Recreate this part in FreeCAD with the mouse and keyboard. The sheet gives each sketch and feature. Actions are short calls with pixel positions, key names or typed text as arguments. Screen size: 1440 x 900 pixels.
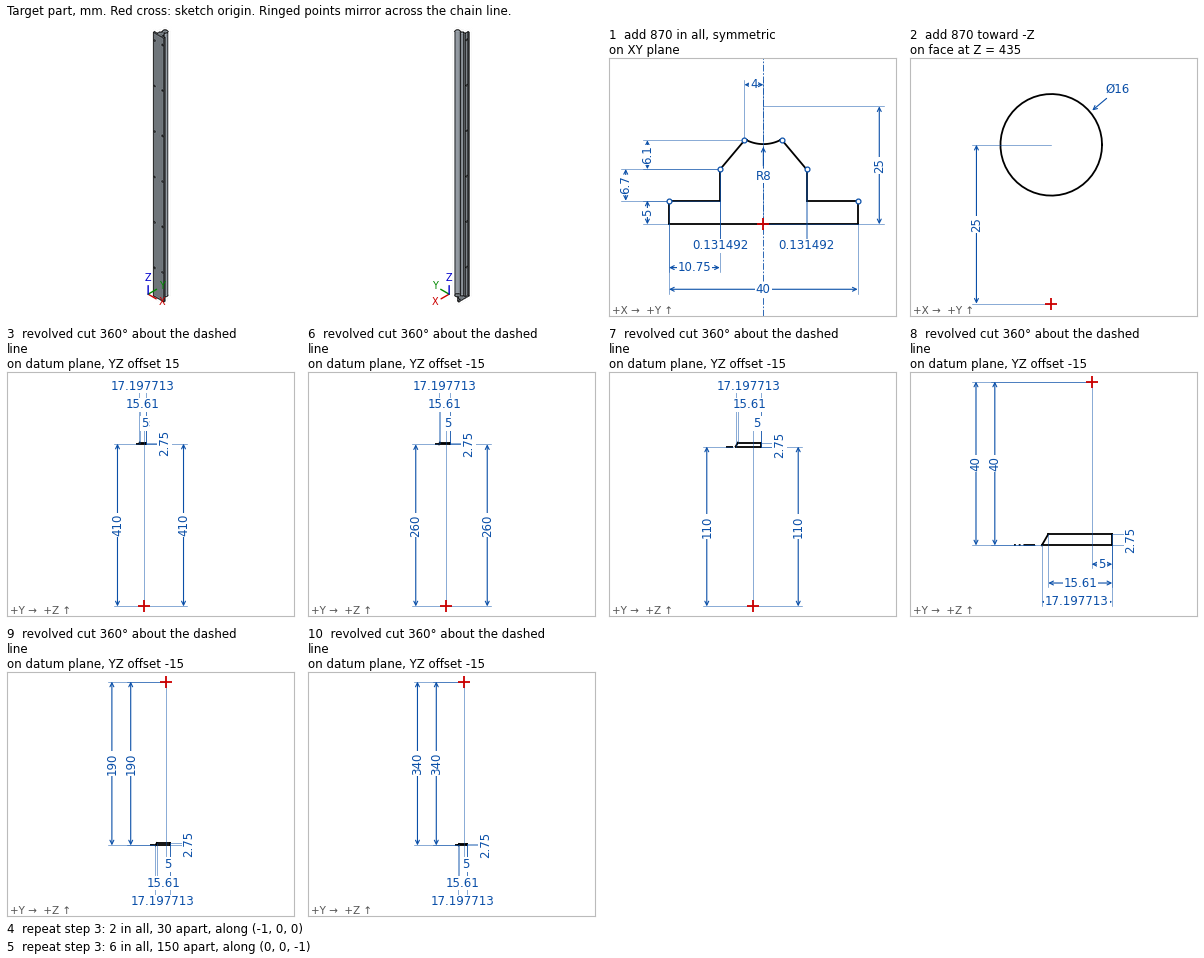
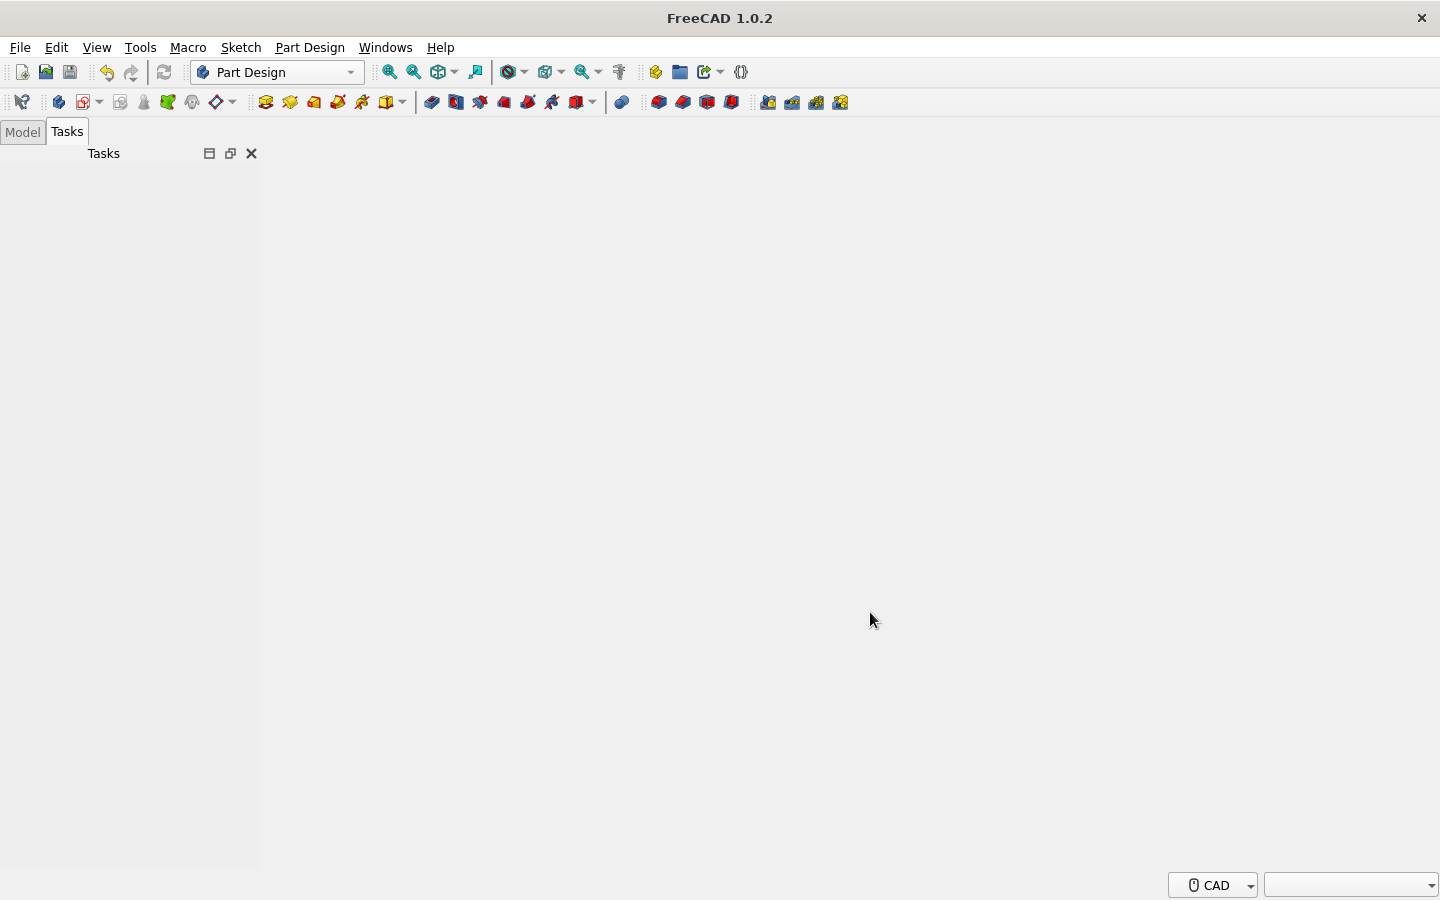
click(22, 72)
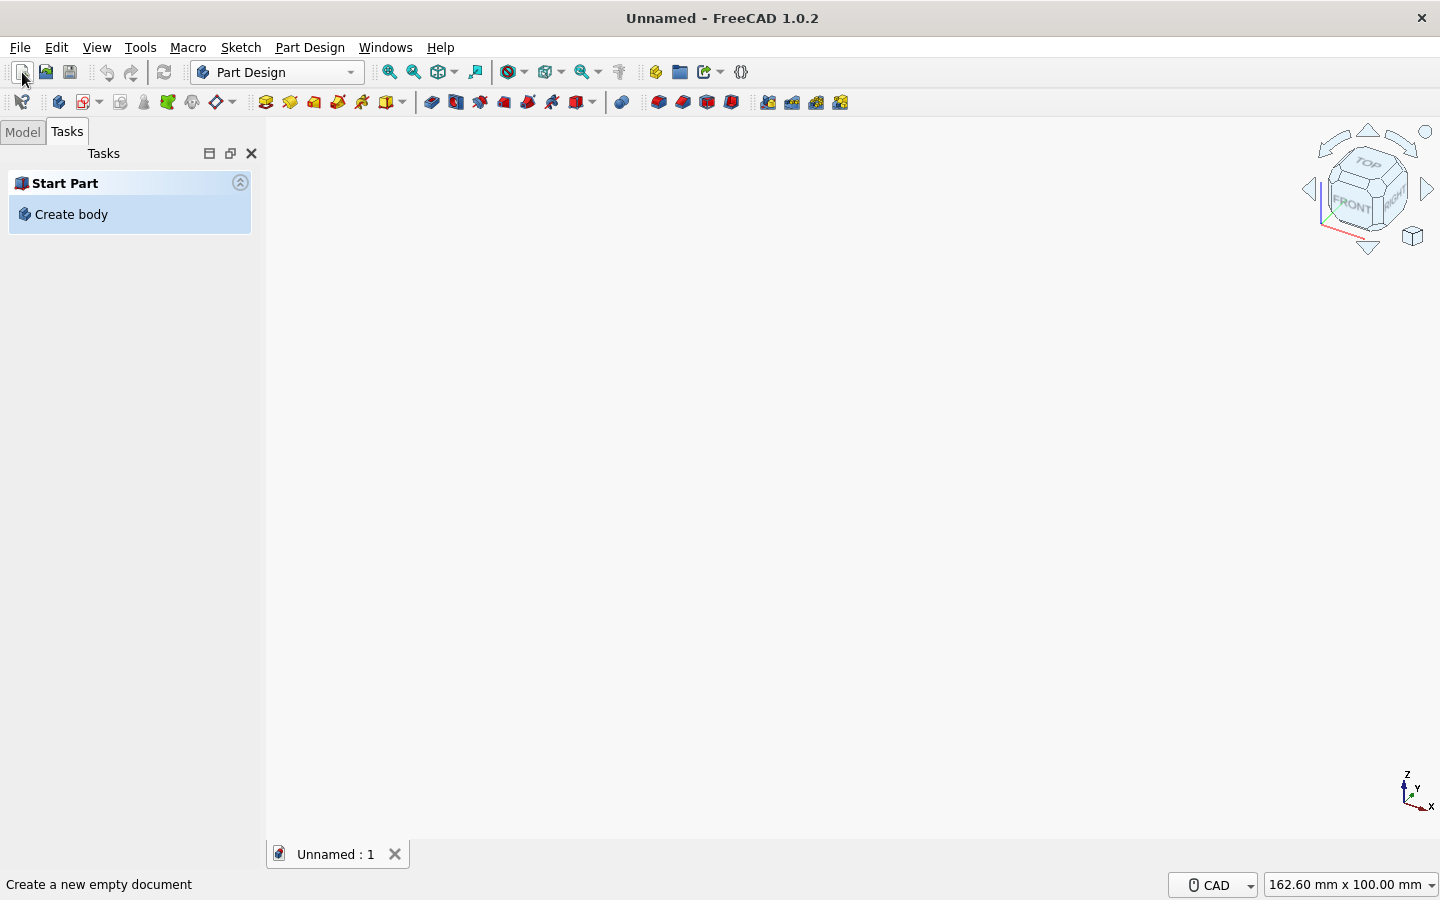
click(84, 102)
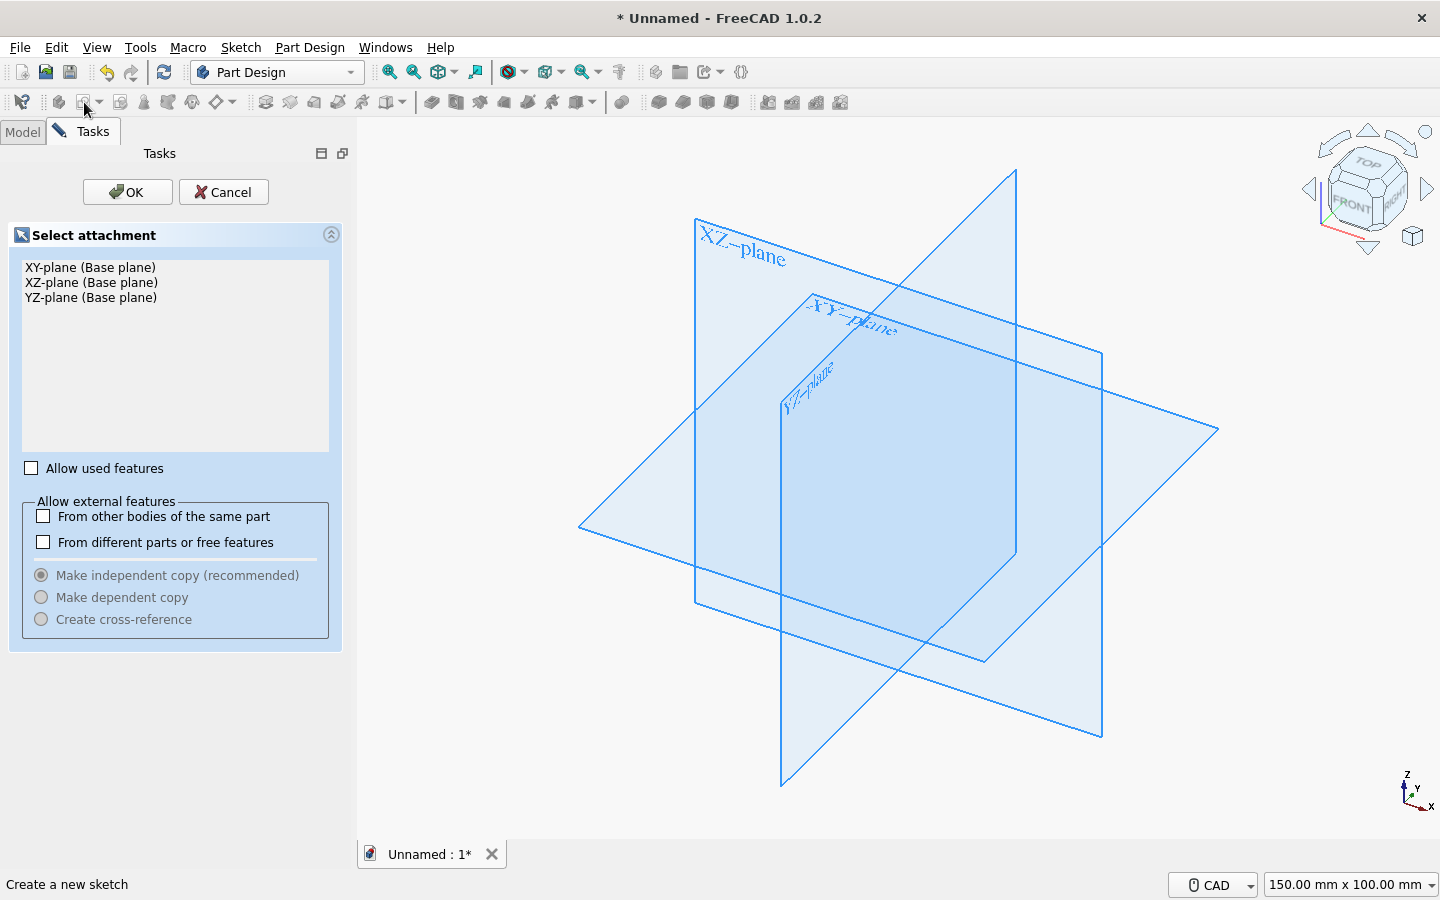
click(82, 268)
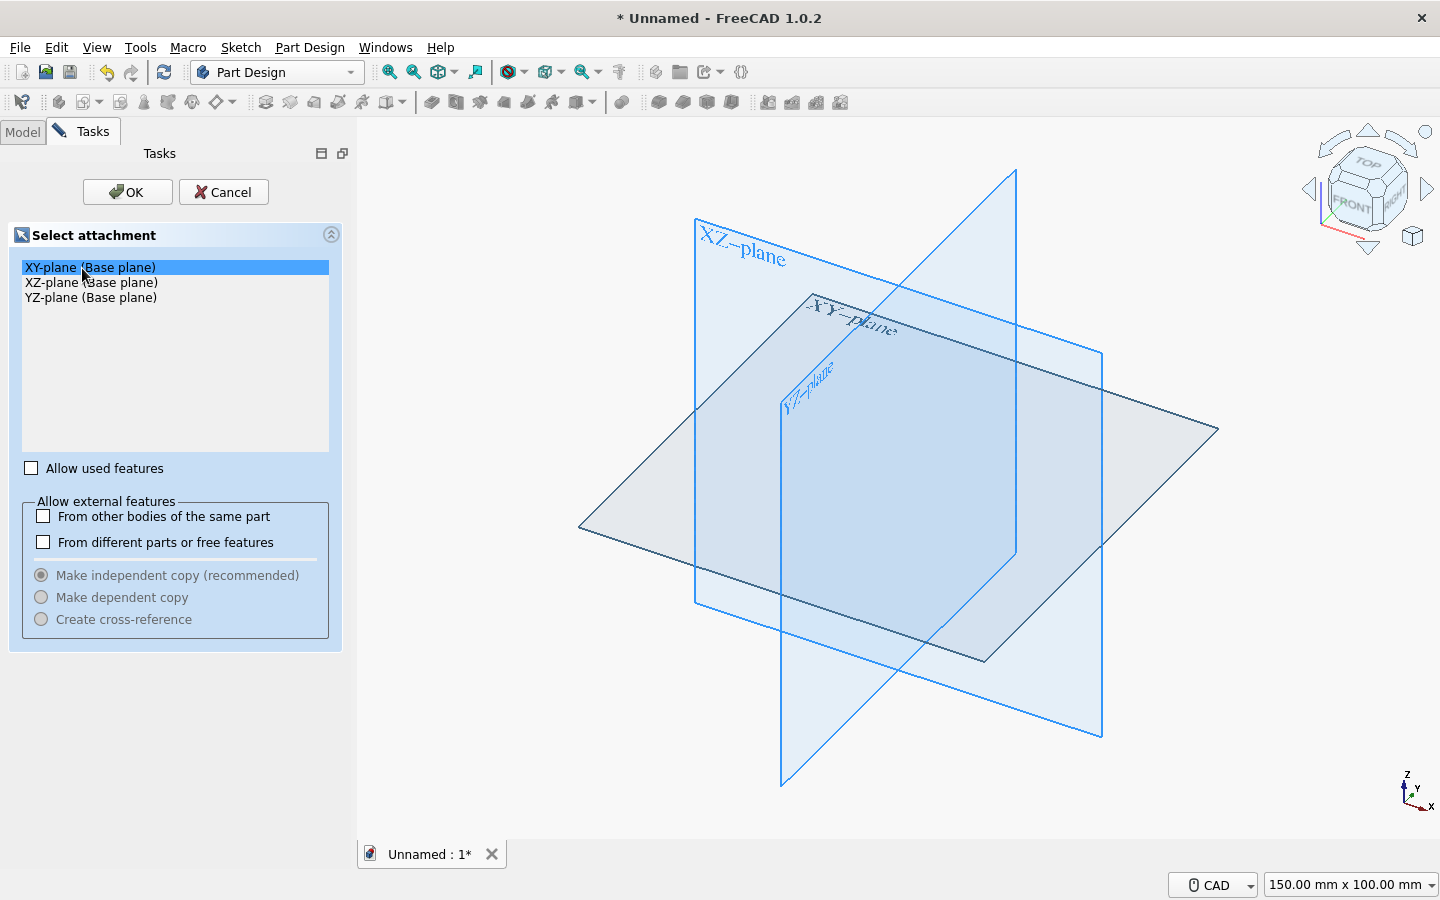
click(128, 192)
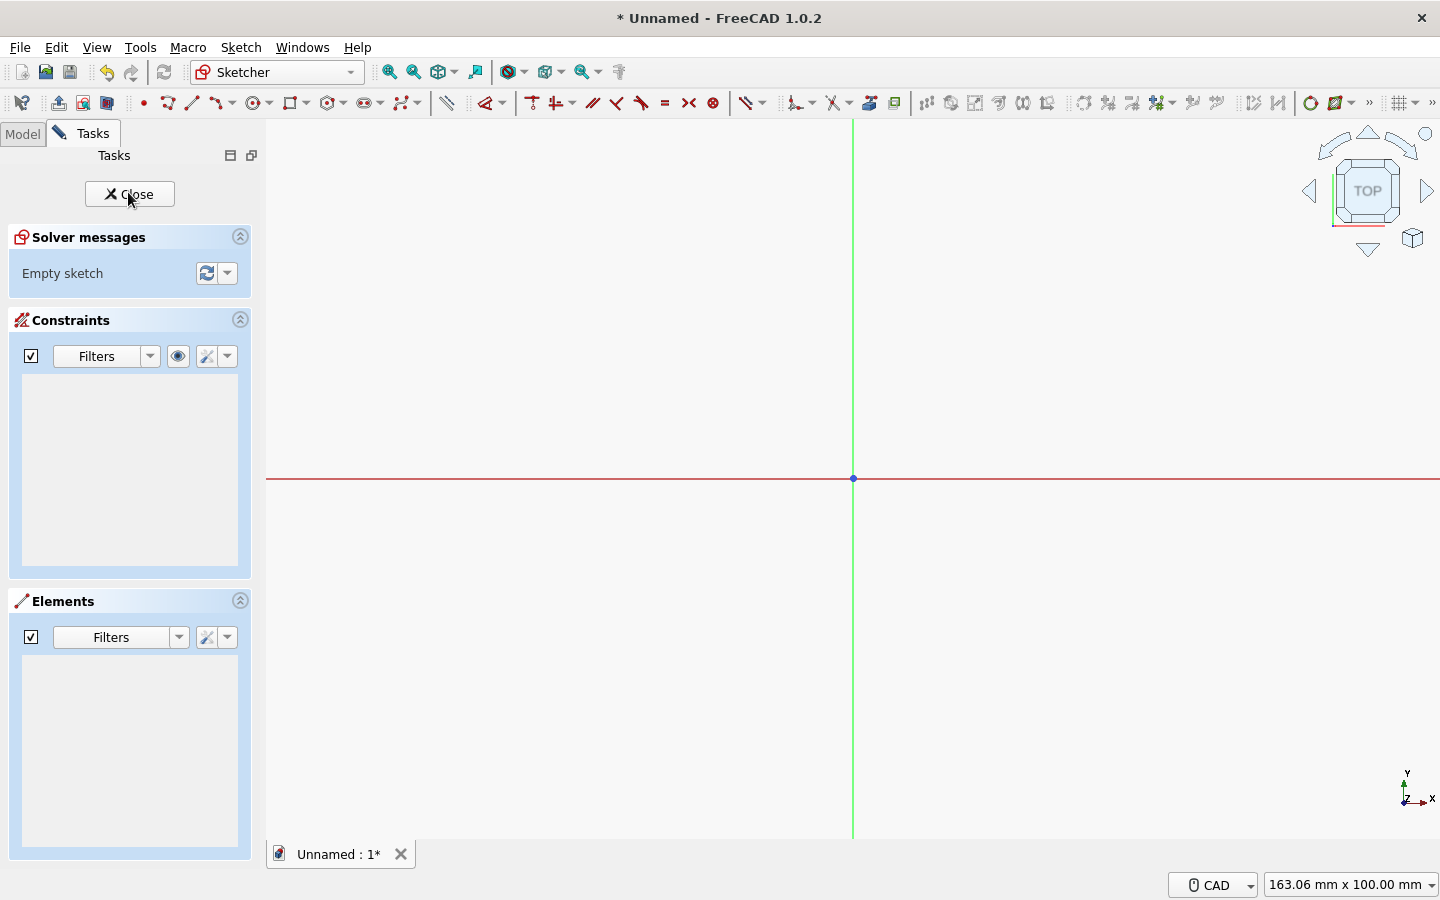
scroll(909, 363, up, 4)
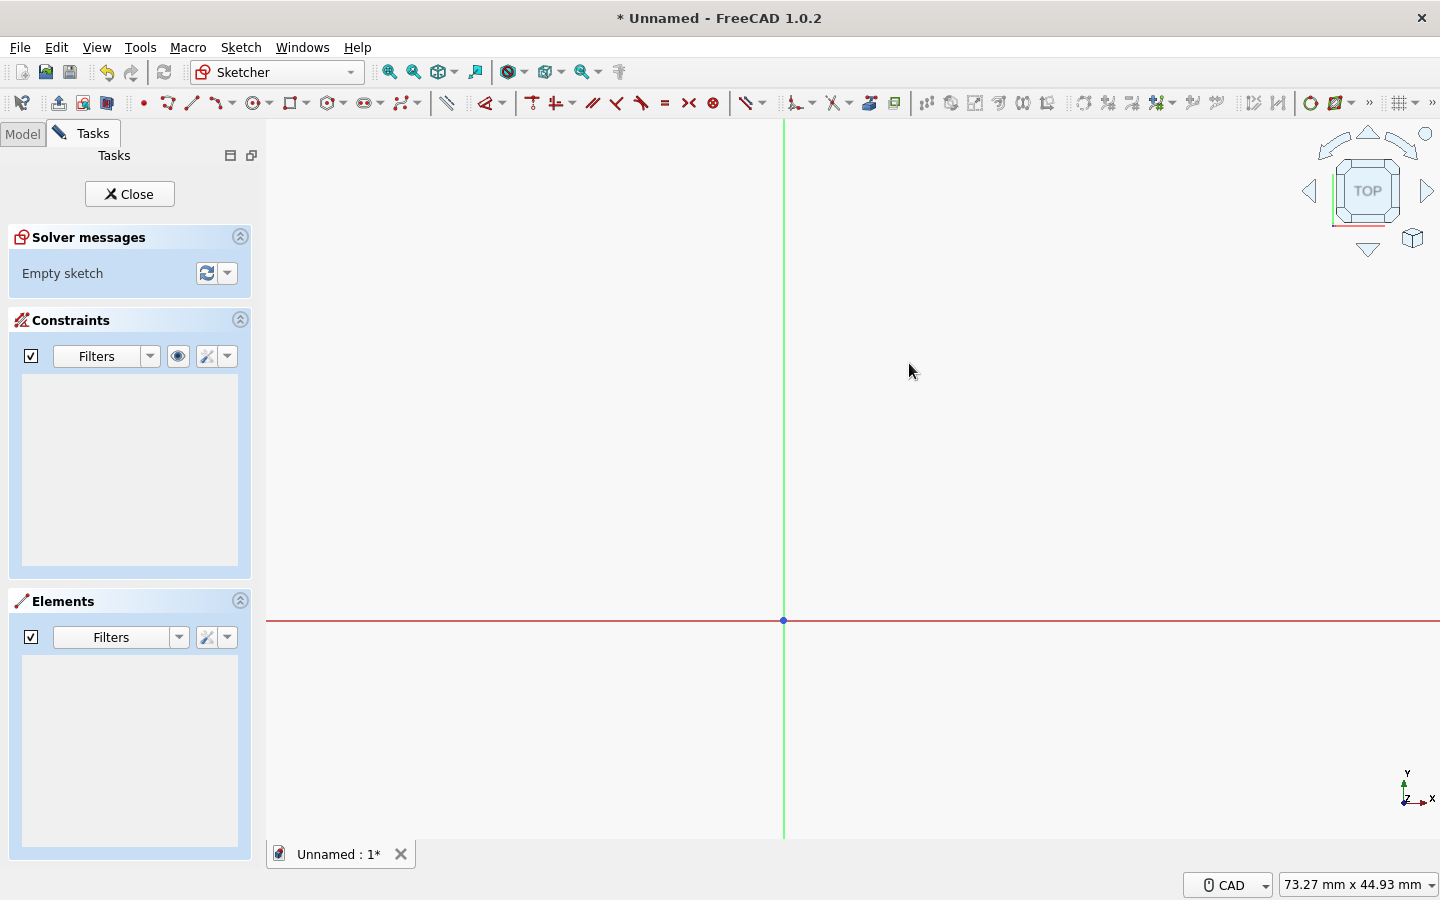
click(168, 104)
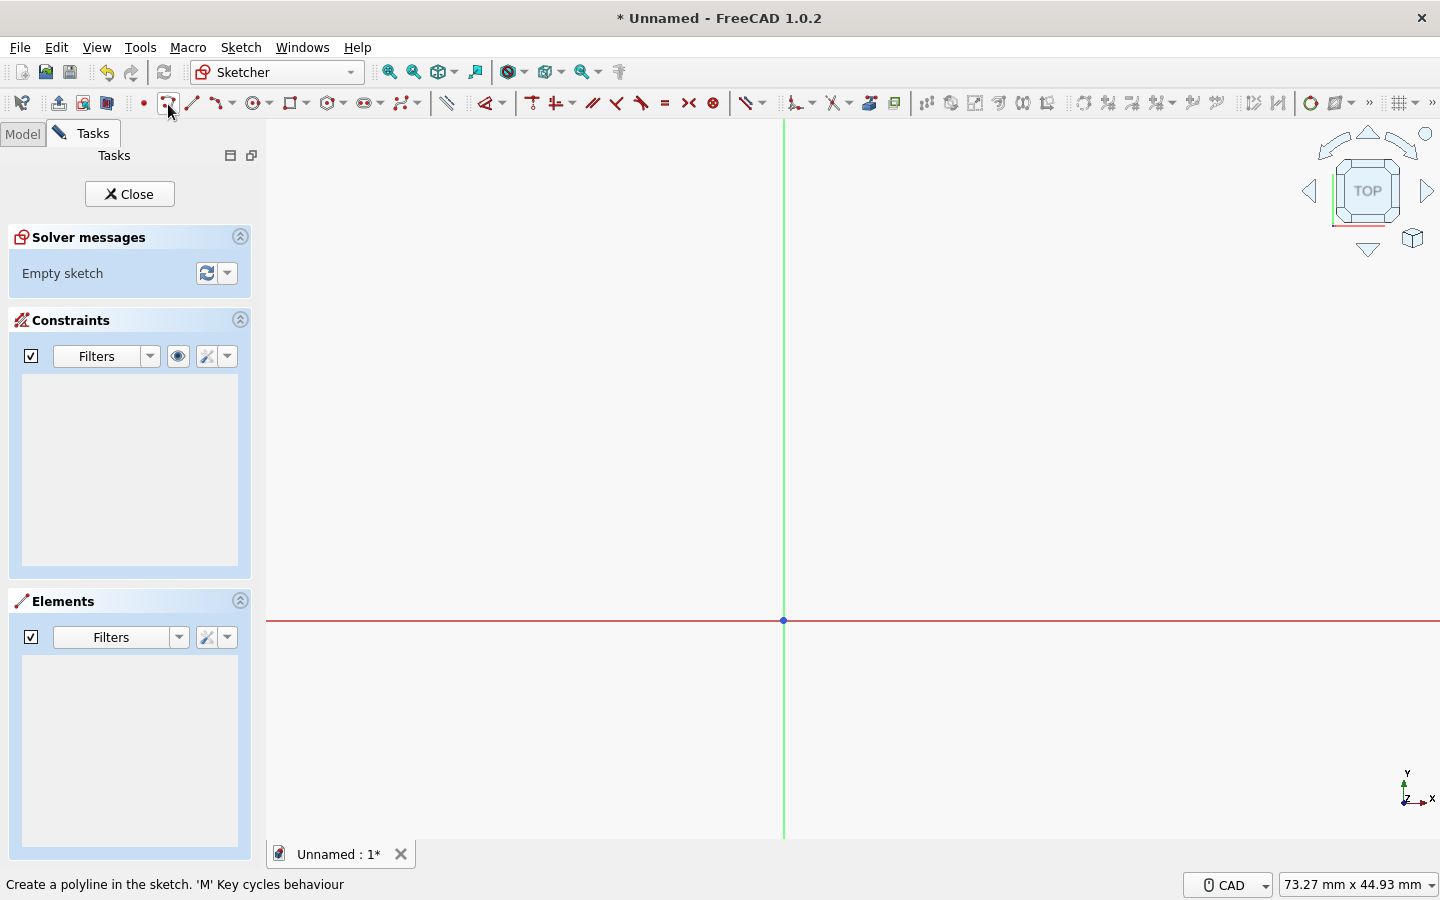
click(728, 336)